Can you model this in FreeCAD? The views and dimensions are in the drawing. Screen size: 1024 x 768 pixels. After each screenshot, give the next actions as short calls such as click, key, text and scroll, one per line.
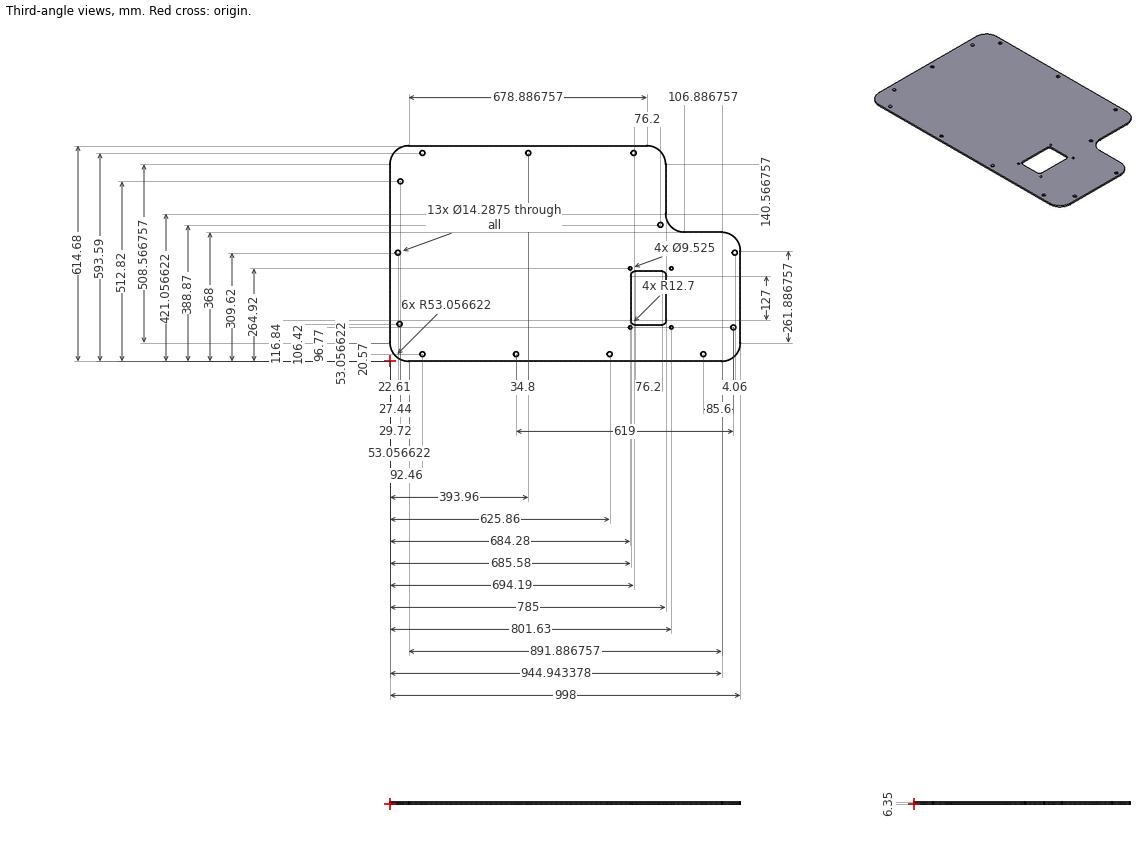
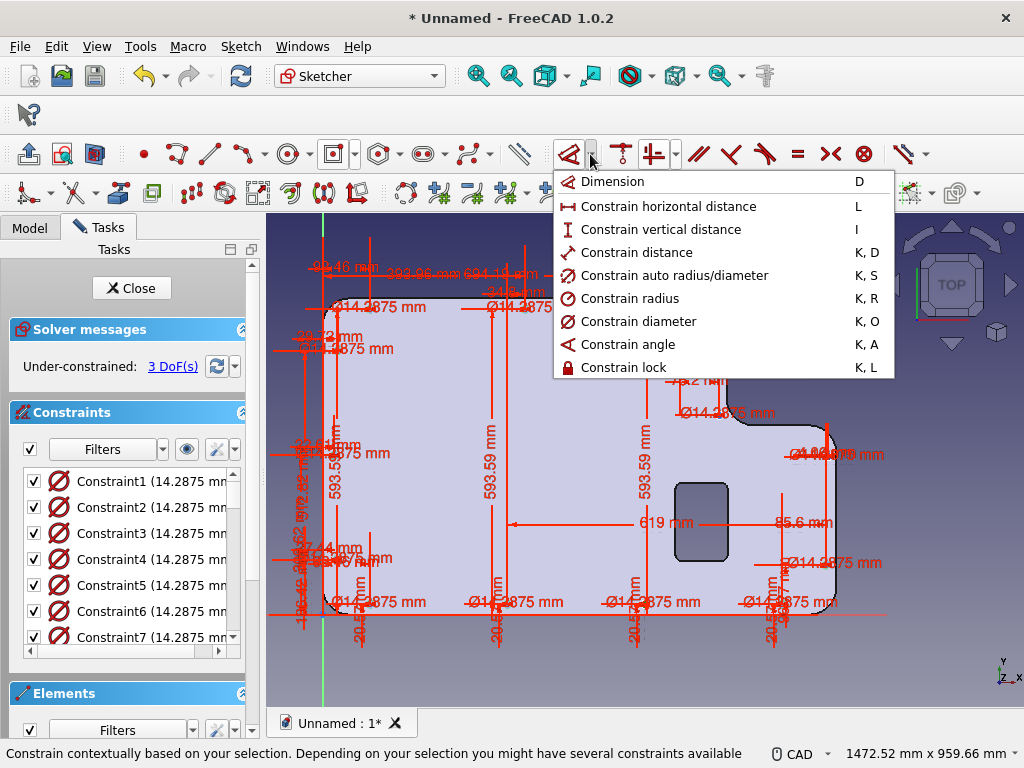
click(724, 206)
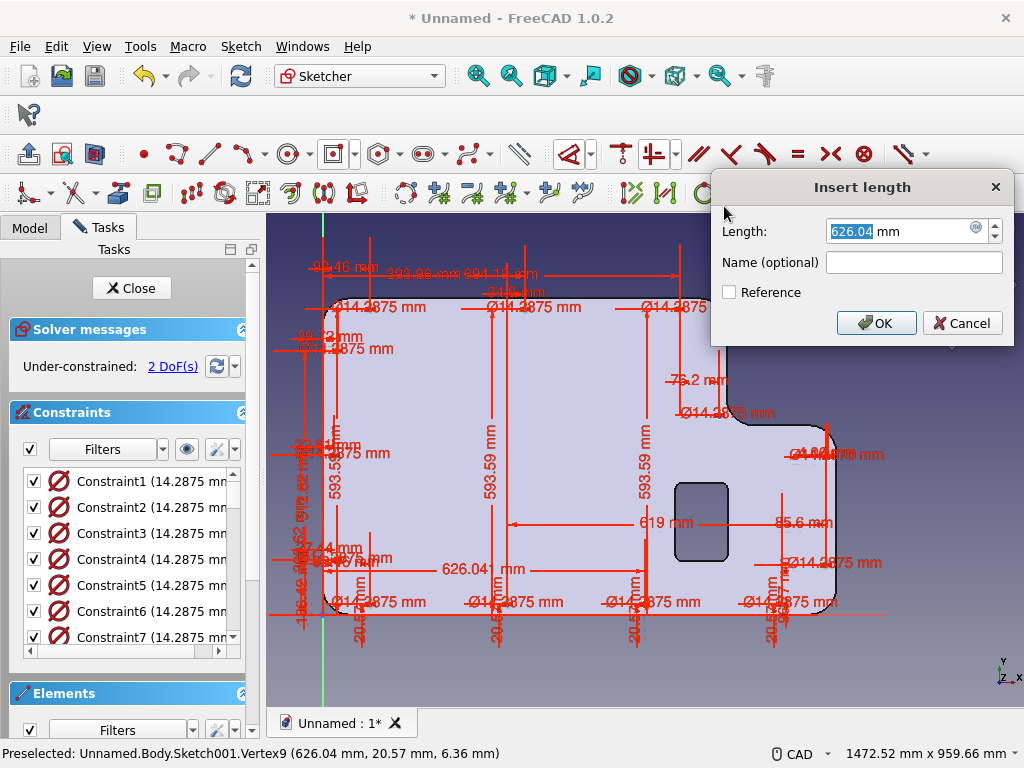
text(625.86)
key(Return)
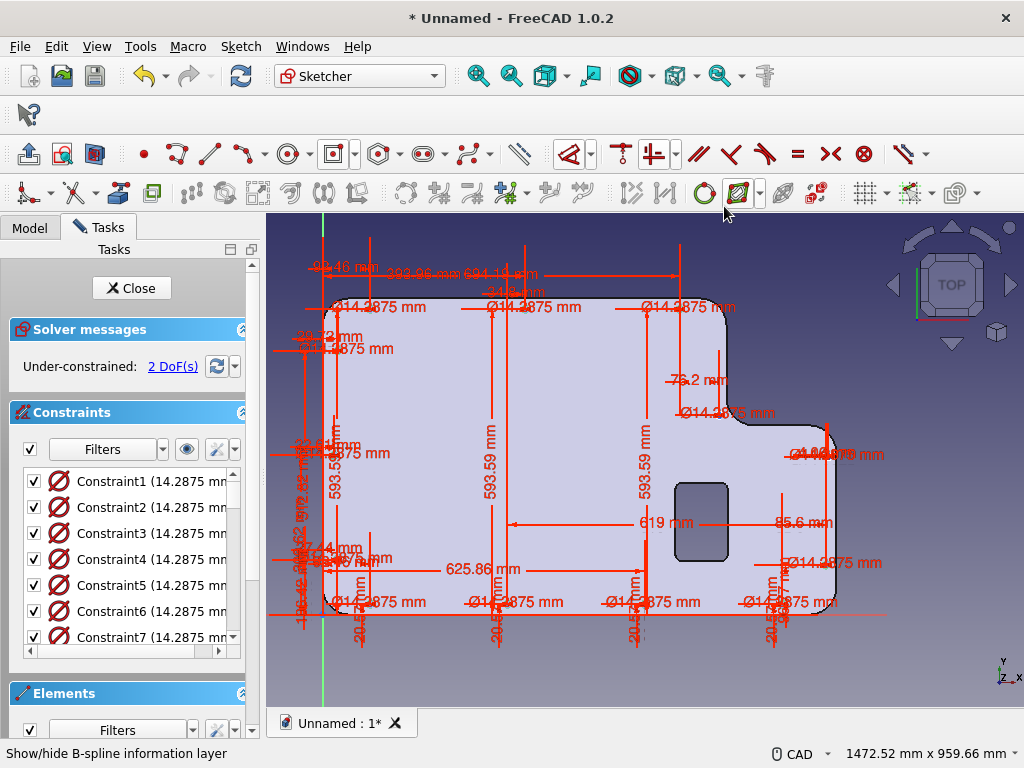
click(828, 457)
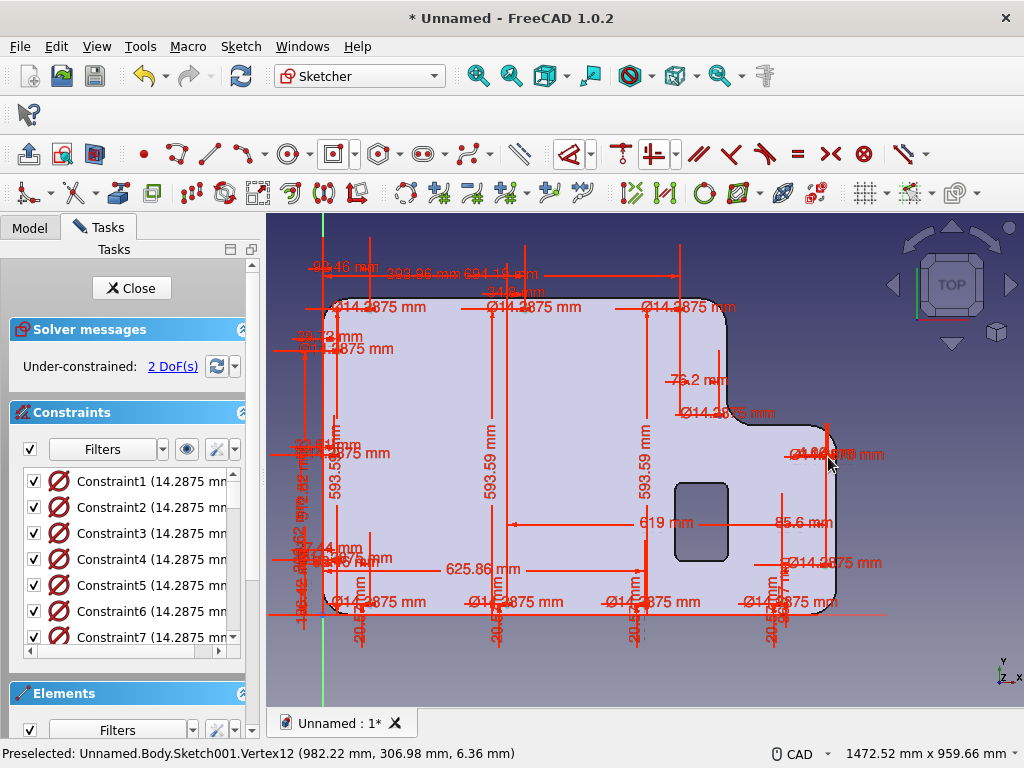
click(590, 154)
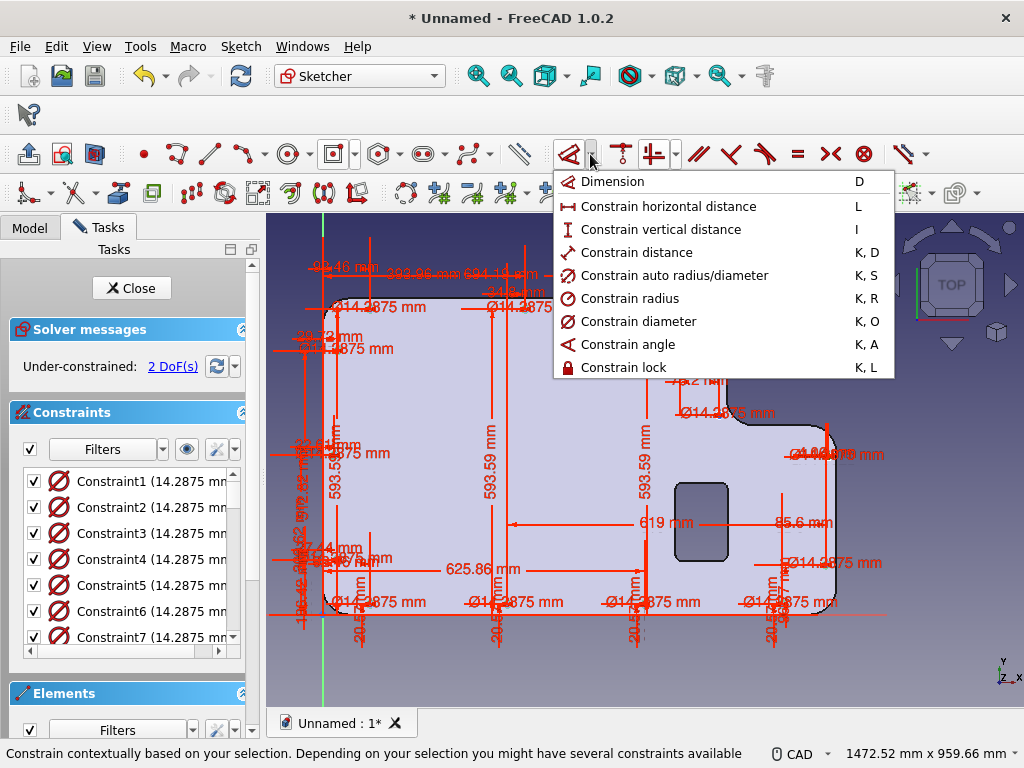
click(724, 230)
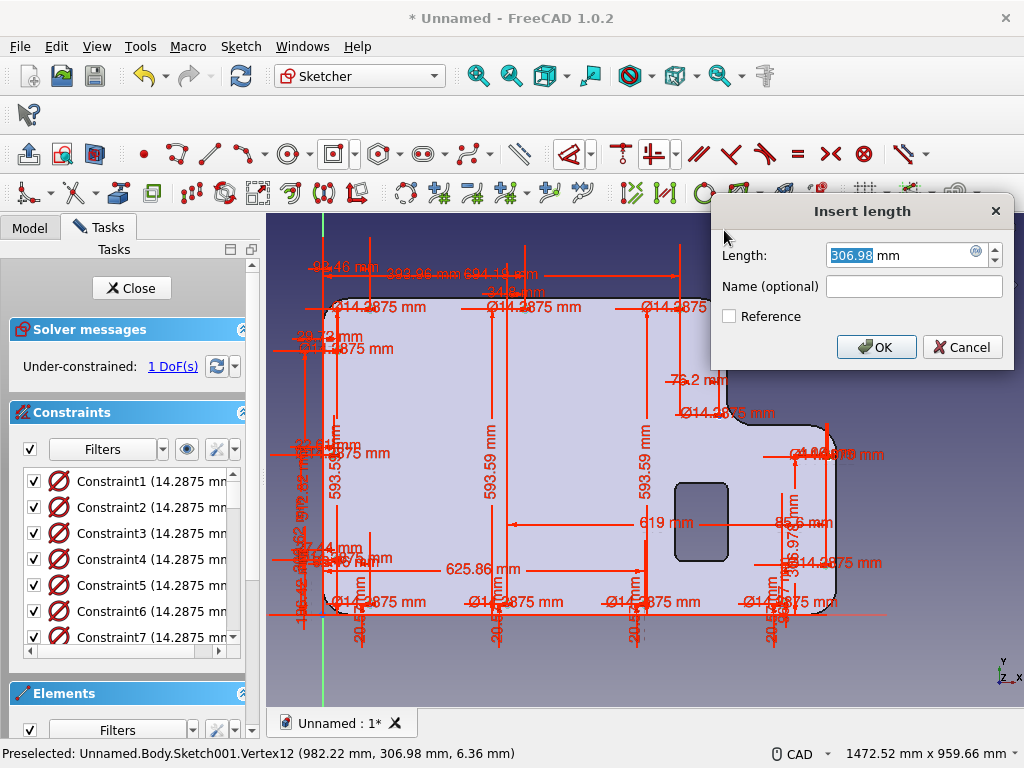
text(309.62)
key(Return)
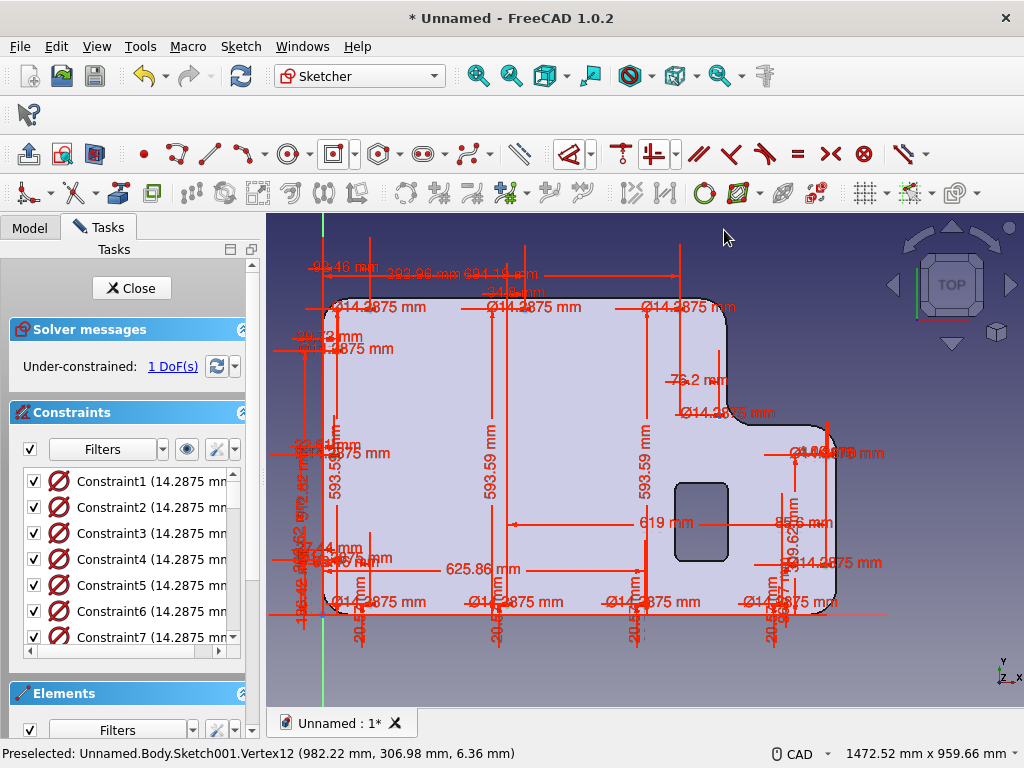
click(719, 415)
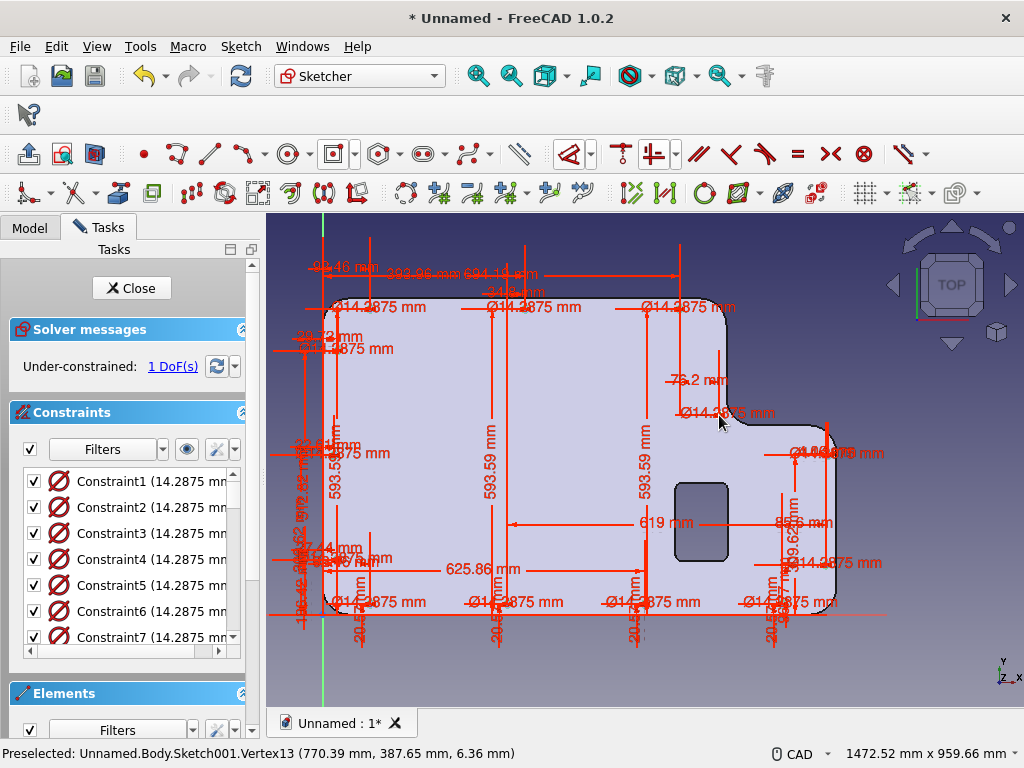
click(590, 154)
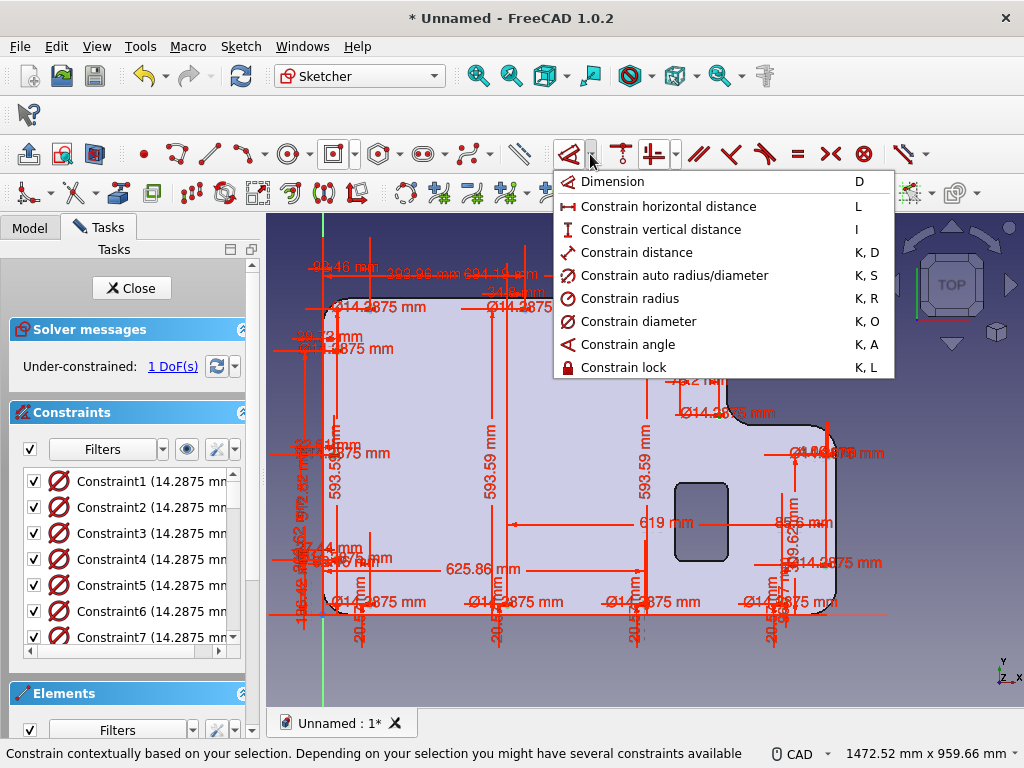
click(724, 230)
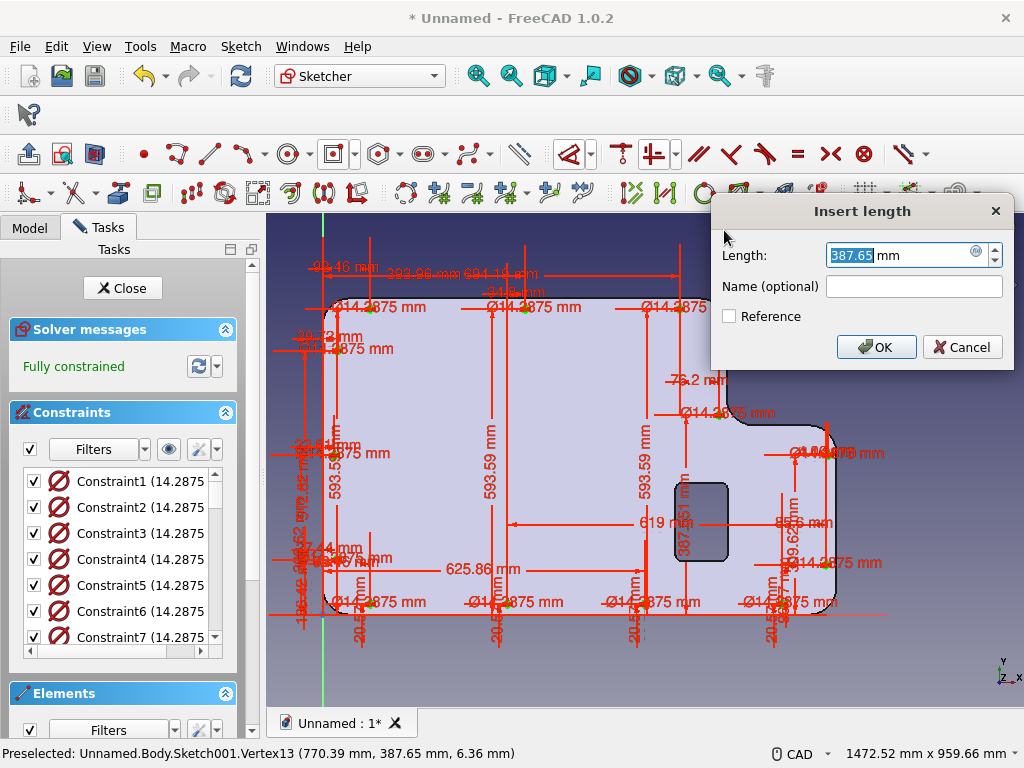
text(388.87)
key(Return)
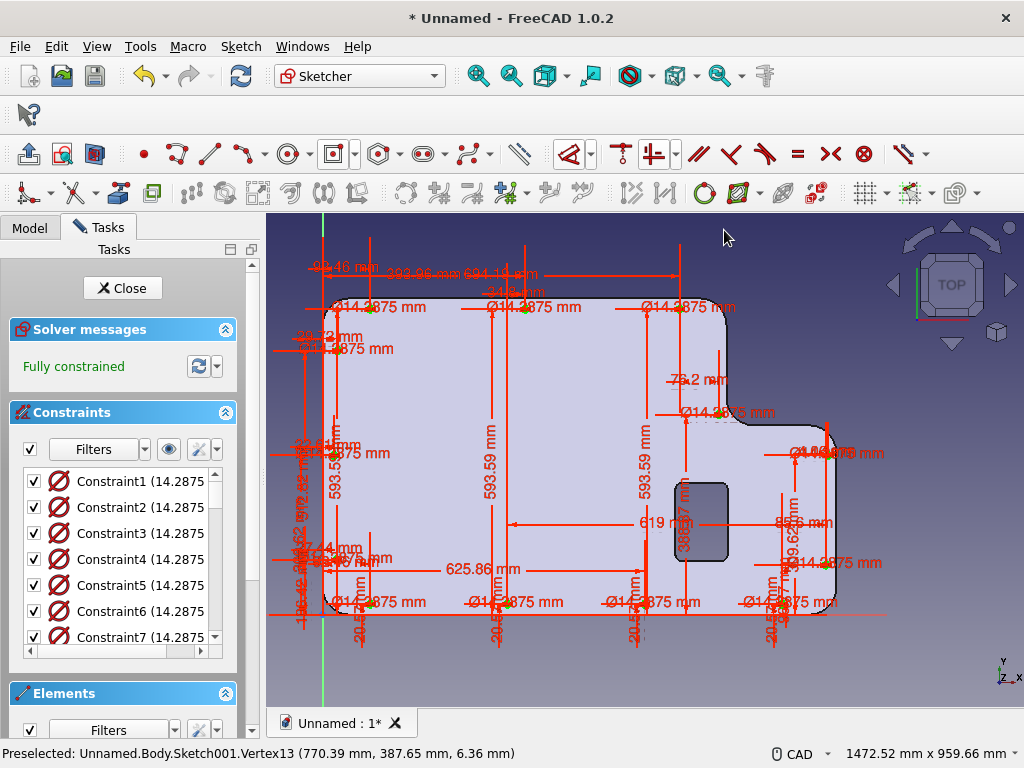
click(123, 288)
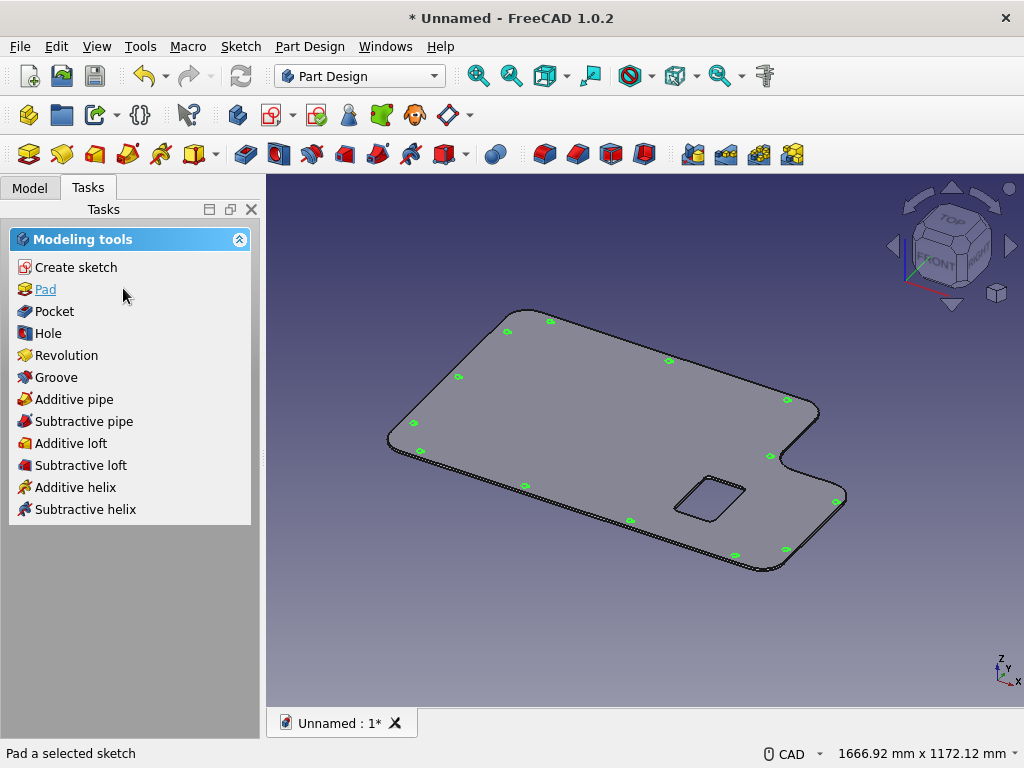
click(279, 154)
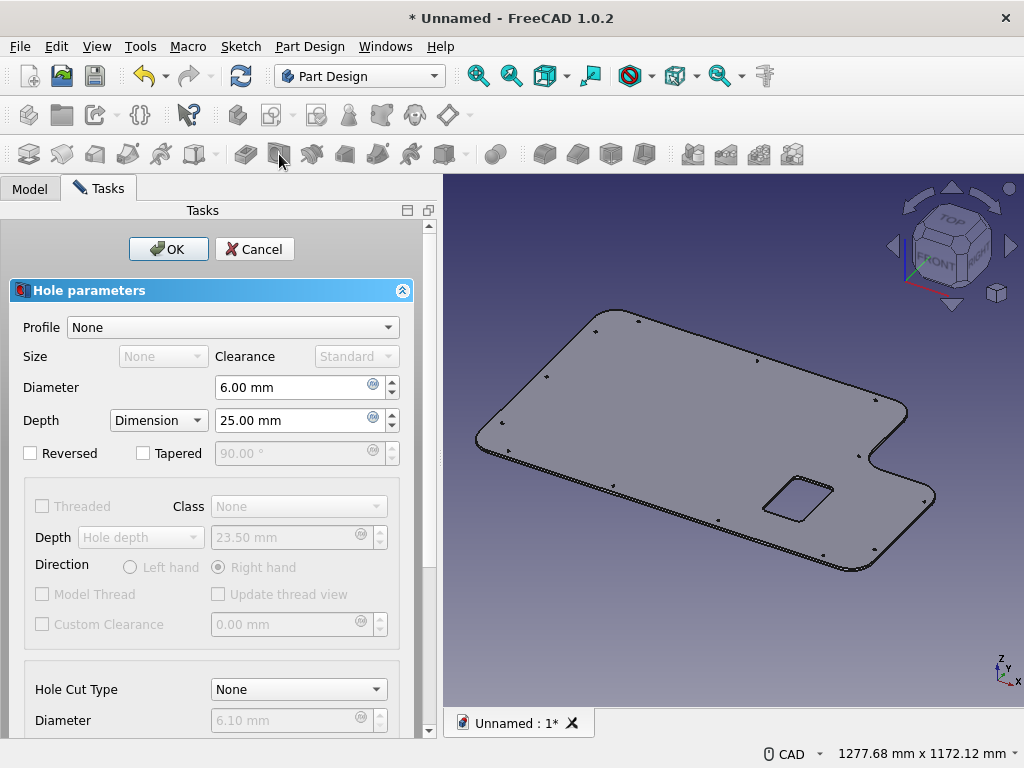
triple_click(300, 388)